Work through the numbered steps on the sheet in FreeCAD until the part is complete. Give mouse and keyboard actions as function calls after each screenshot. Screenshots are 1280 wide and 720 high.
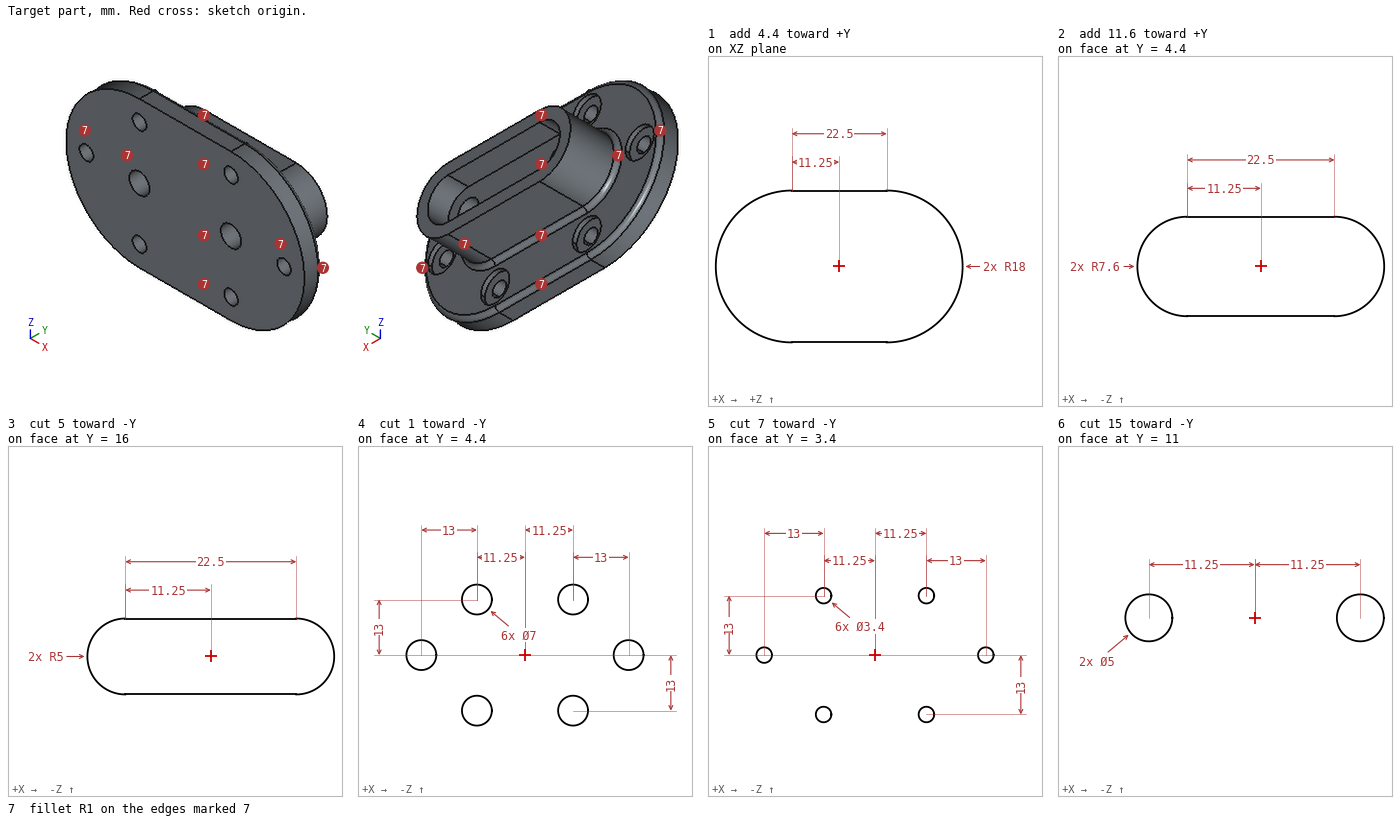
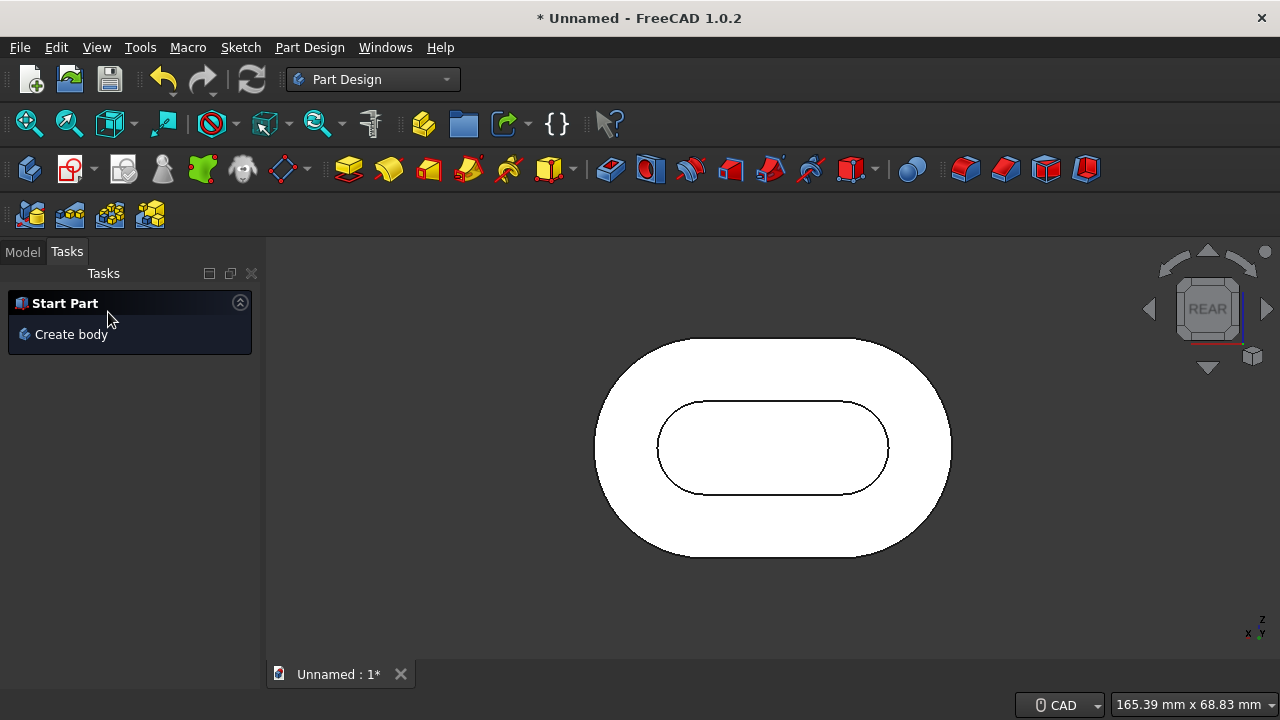
click(707, 447)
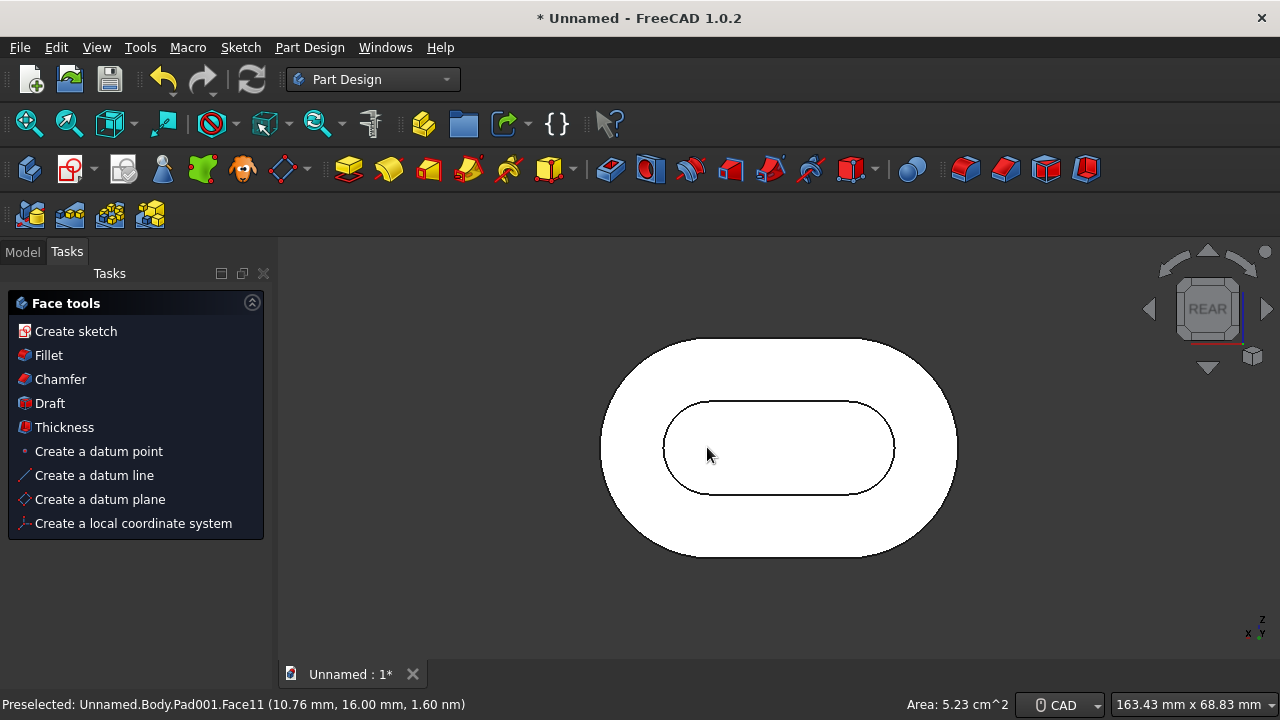
click(70, 170)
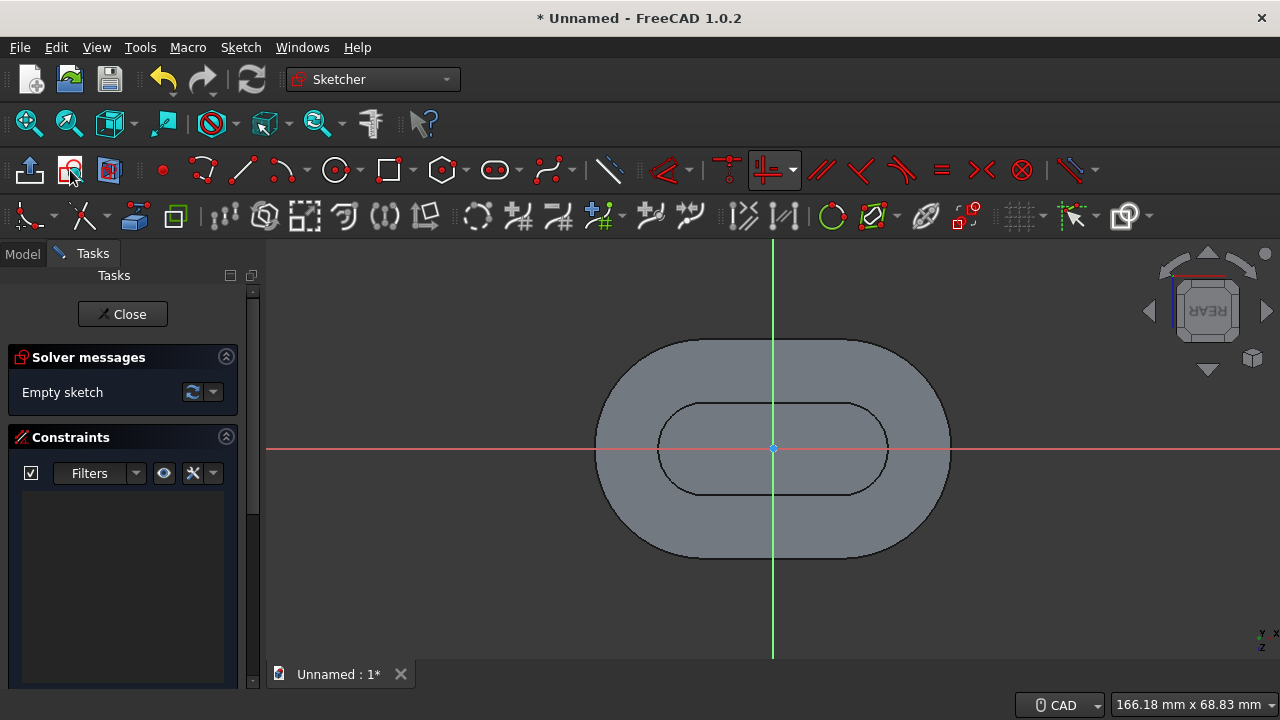
scroll(813, 449, up, 5)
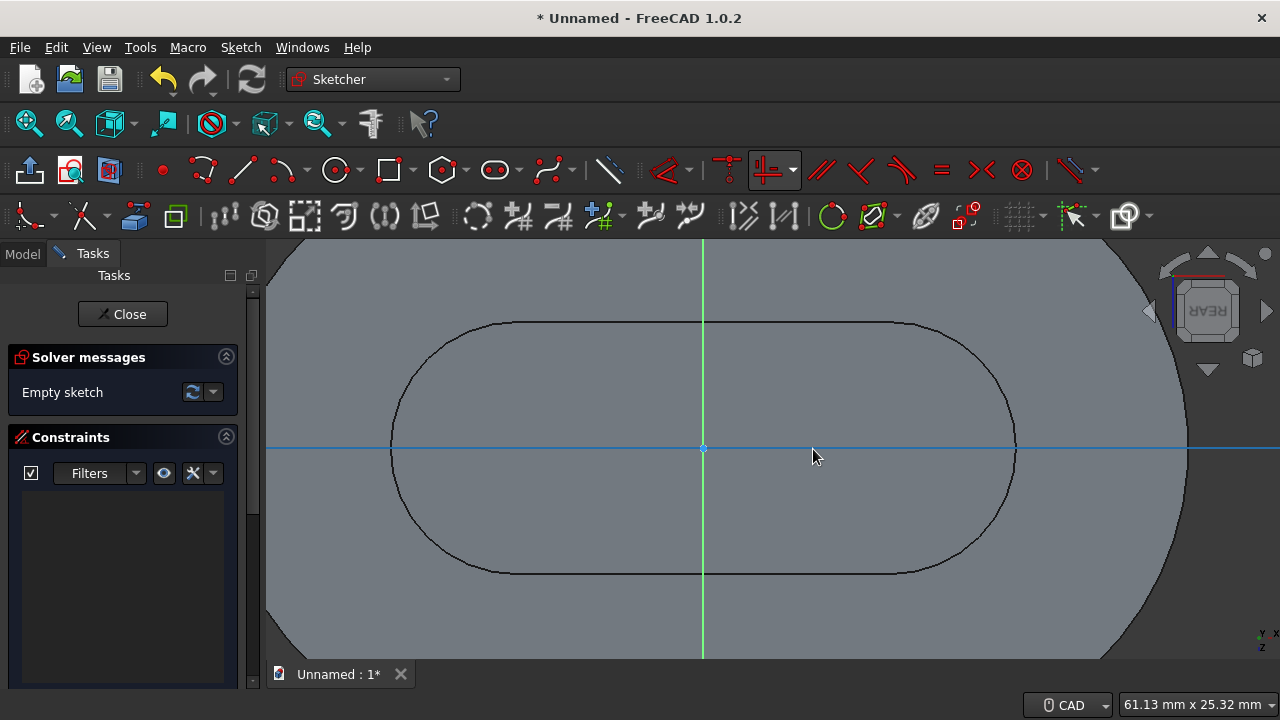
click(496, 170)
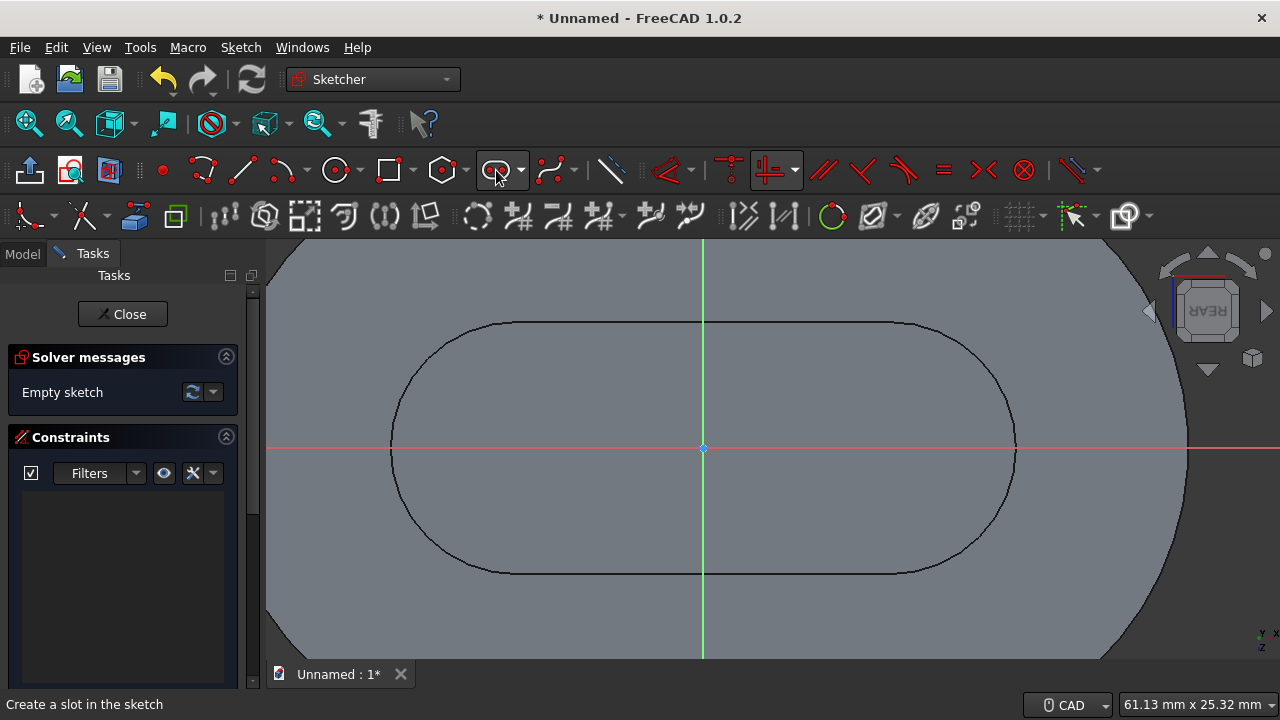
click(517, 448)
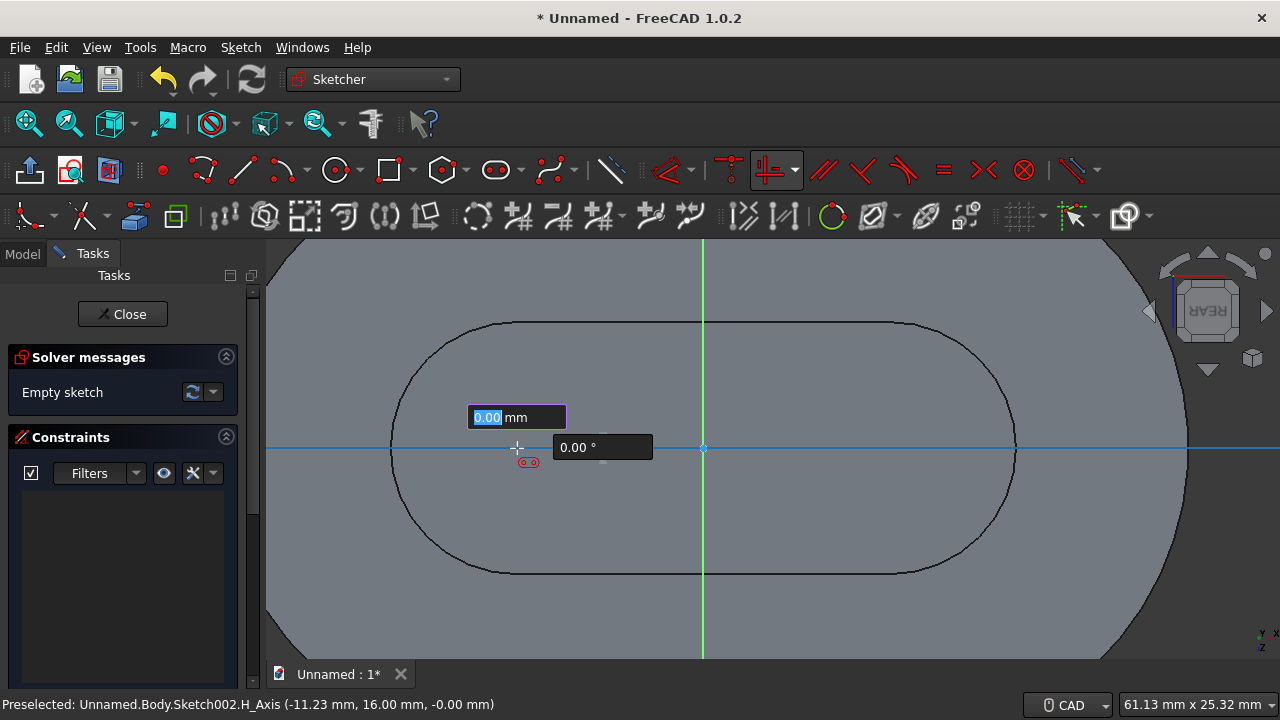
click(890, 439)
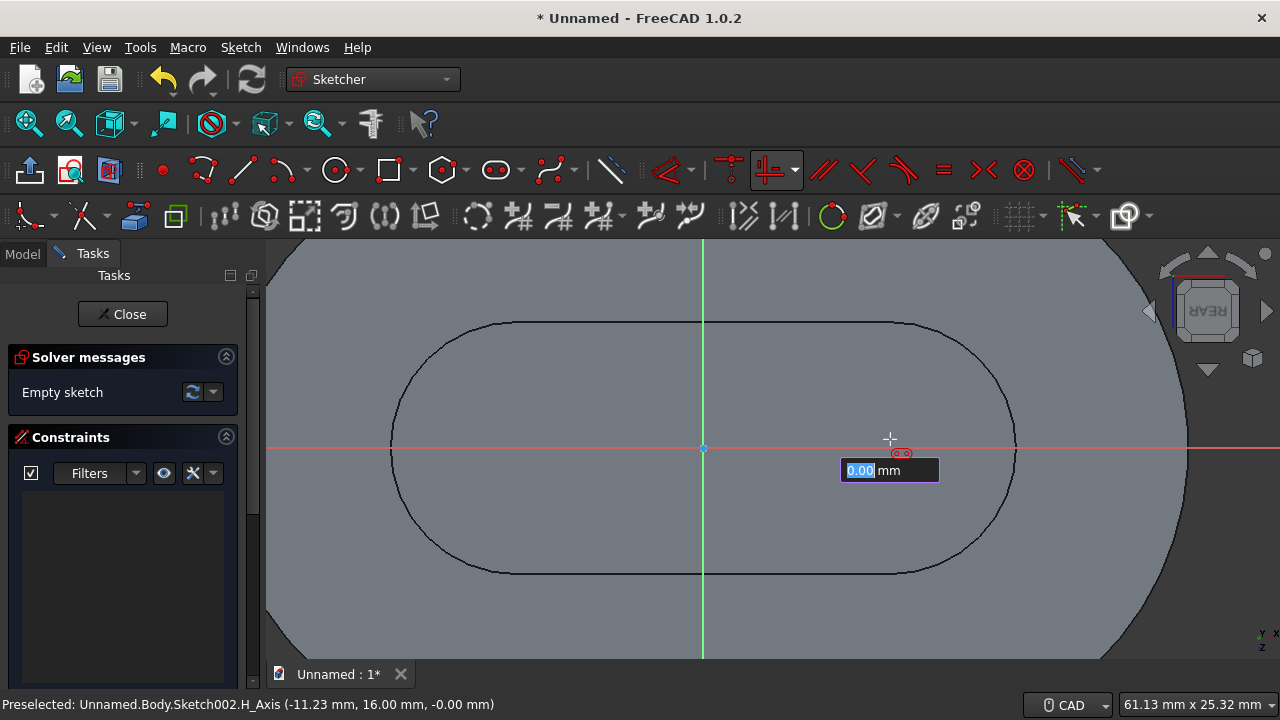
click(759, 365)
key(Escape)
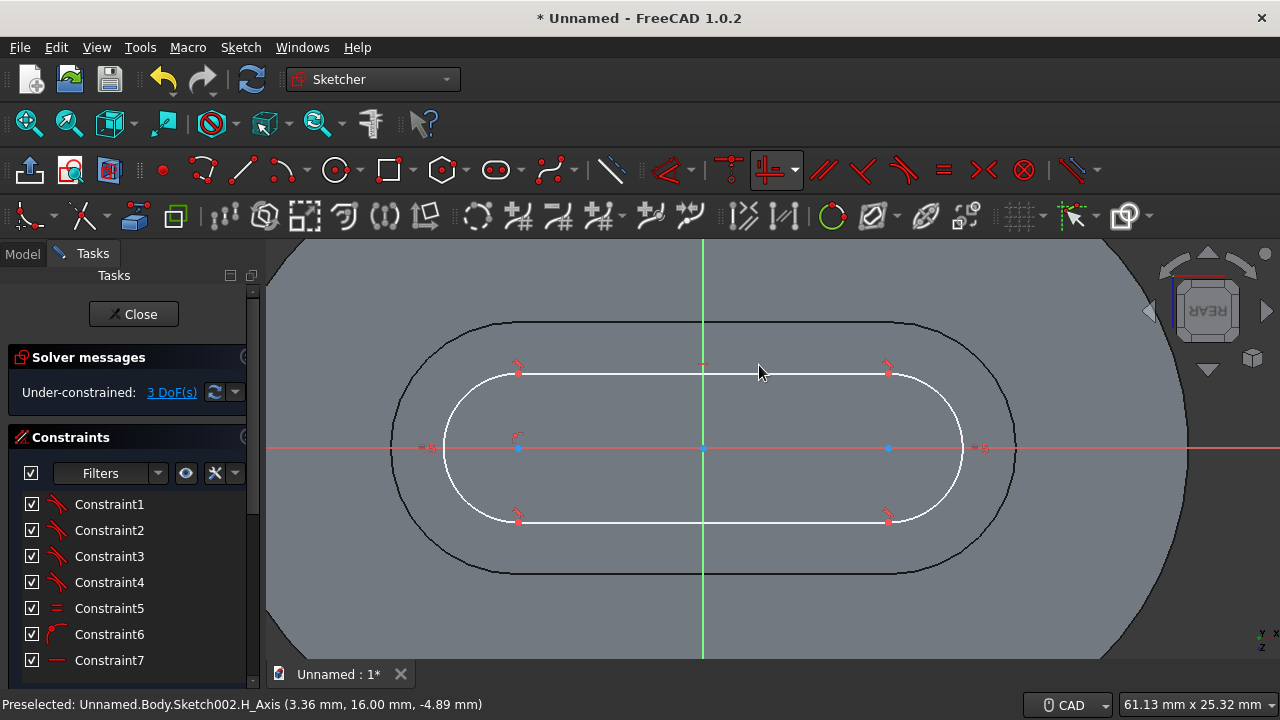
click(666, 170)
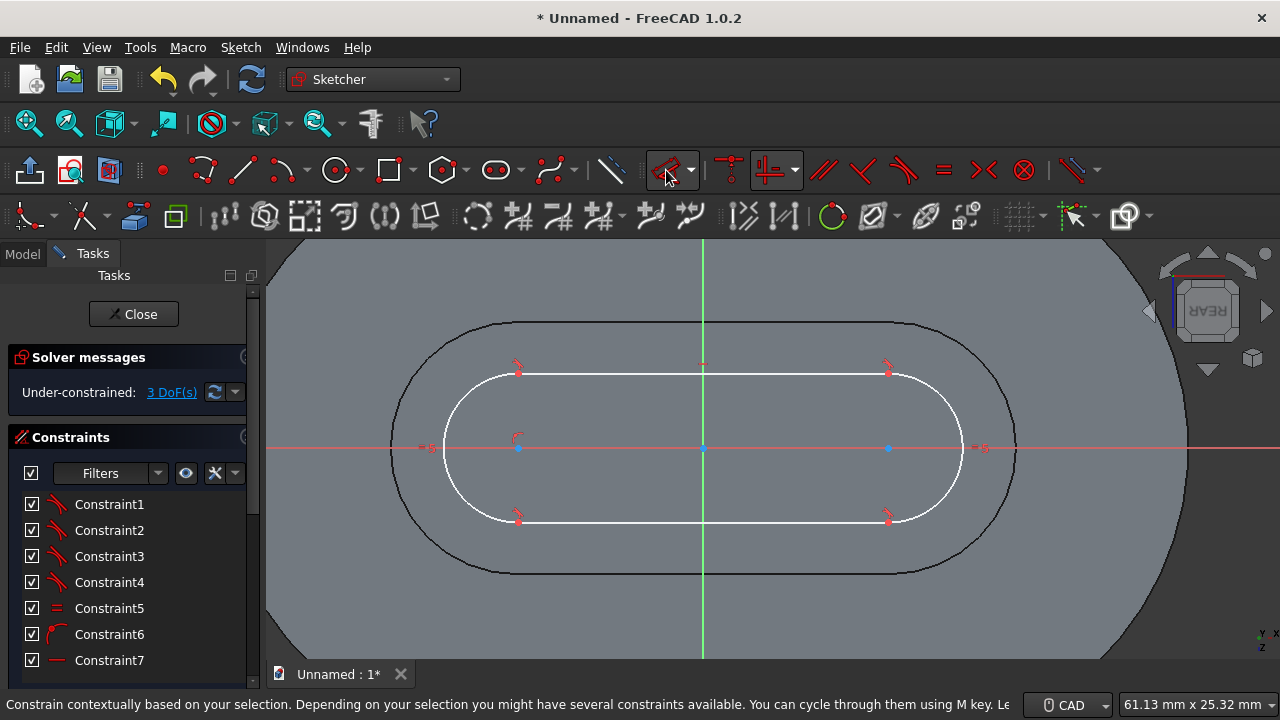
click(458, 404)
click(432, 385)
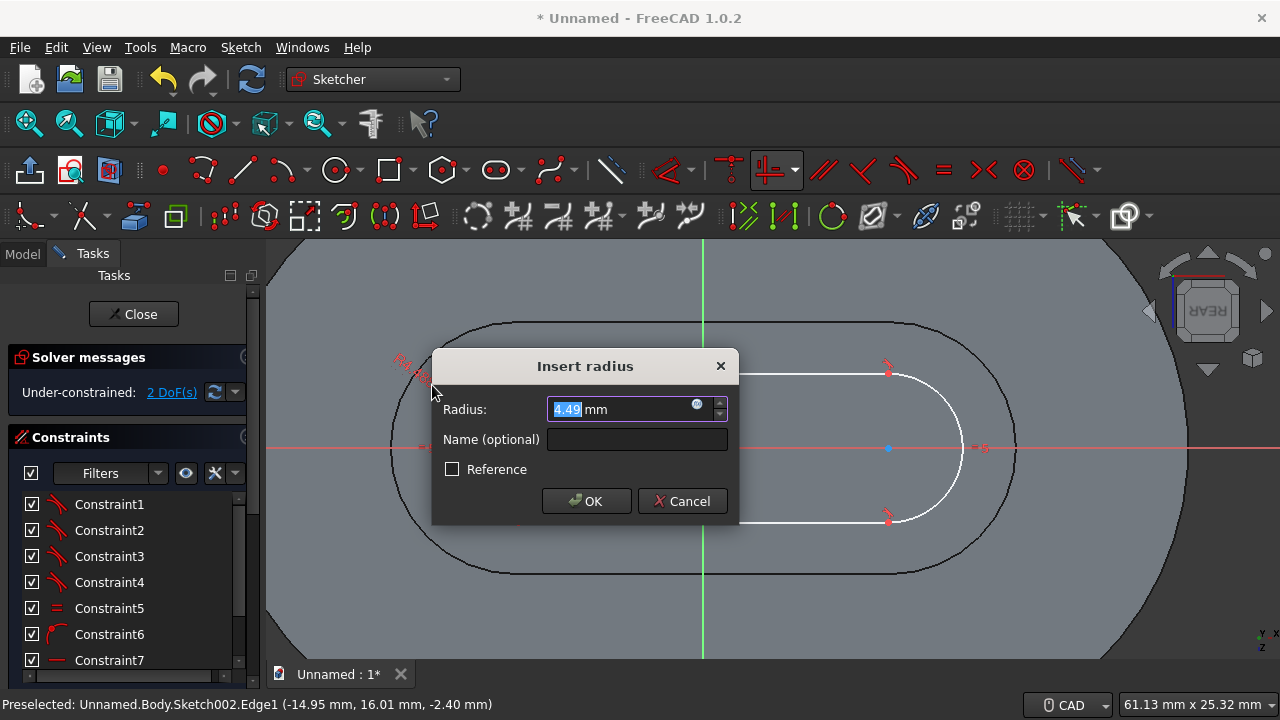
text(5)
key(Return)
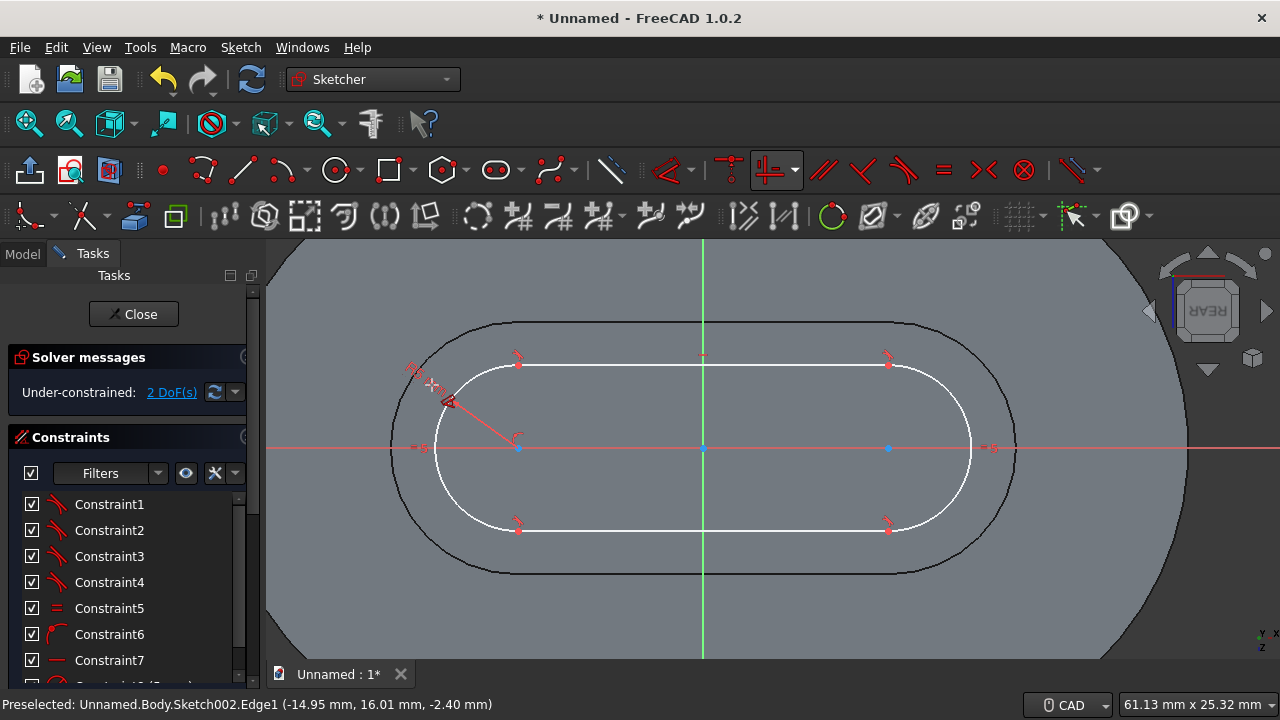
click(629, 365)
click(618, 331)